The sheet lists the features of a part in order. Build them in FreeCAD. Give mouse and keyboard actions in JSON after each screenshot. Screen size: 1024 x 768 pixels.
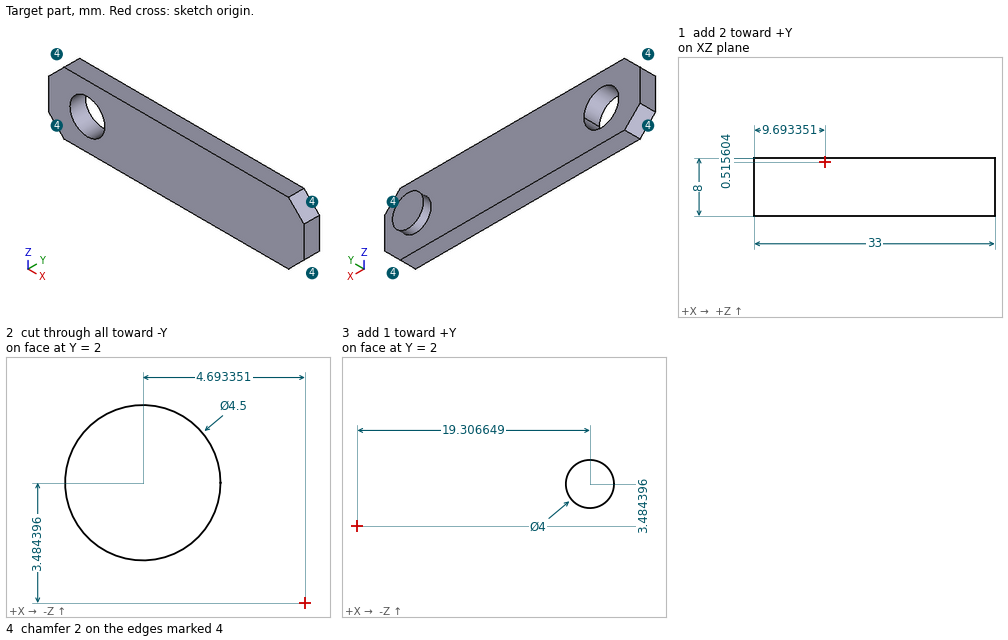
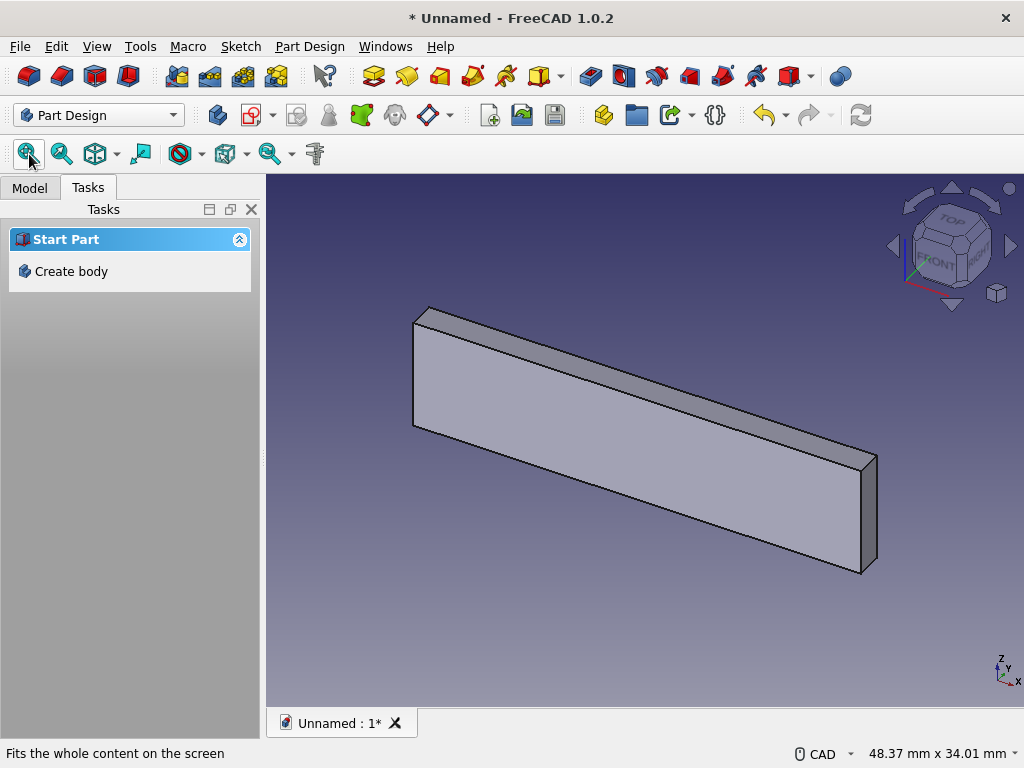
{"action": "key", "text": "4"}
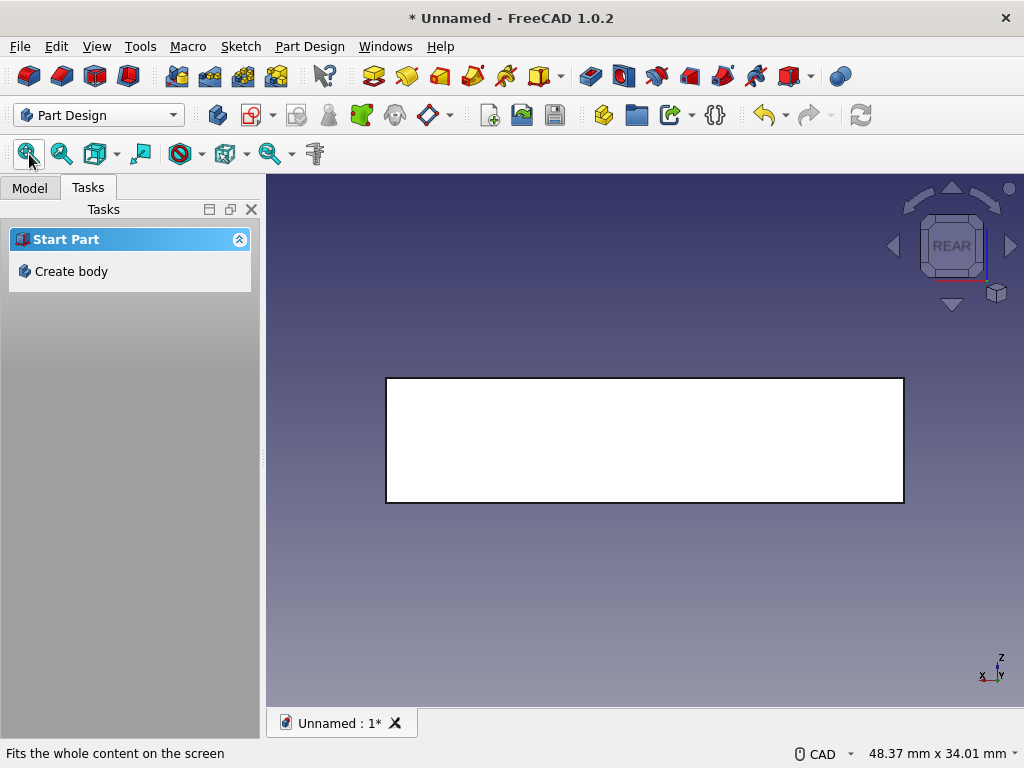
{"action": "left_click", "coordinate": [497, 439]}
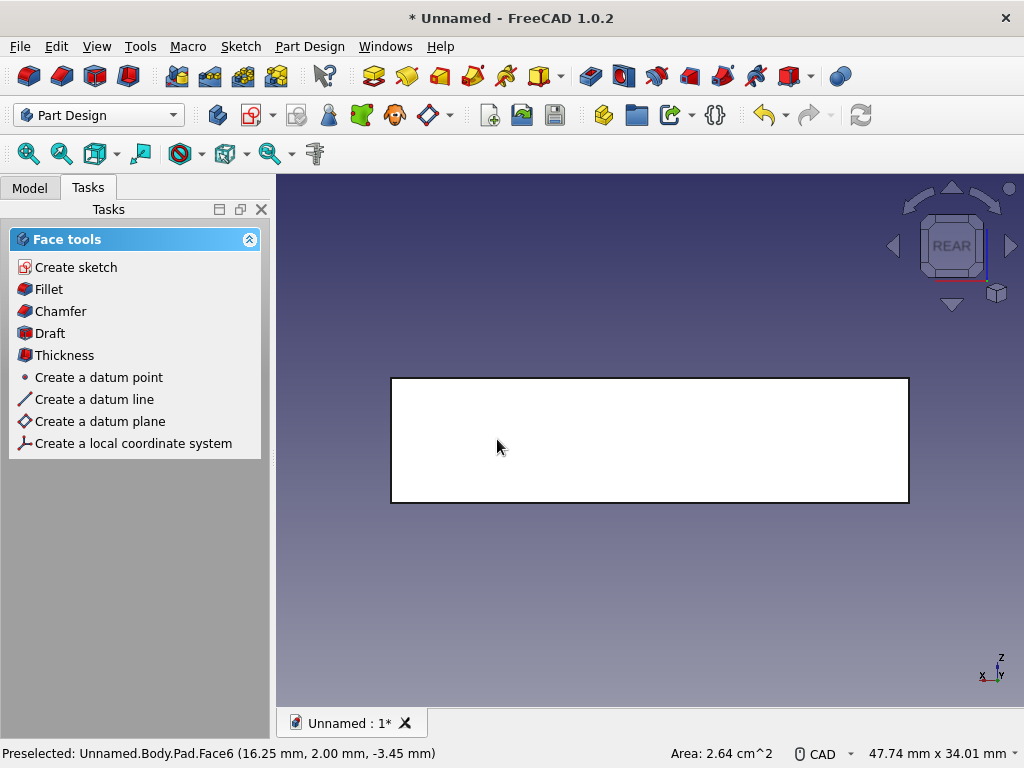
{"action": "left_click", "coordinate": [250, 116]}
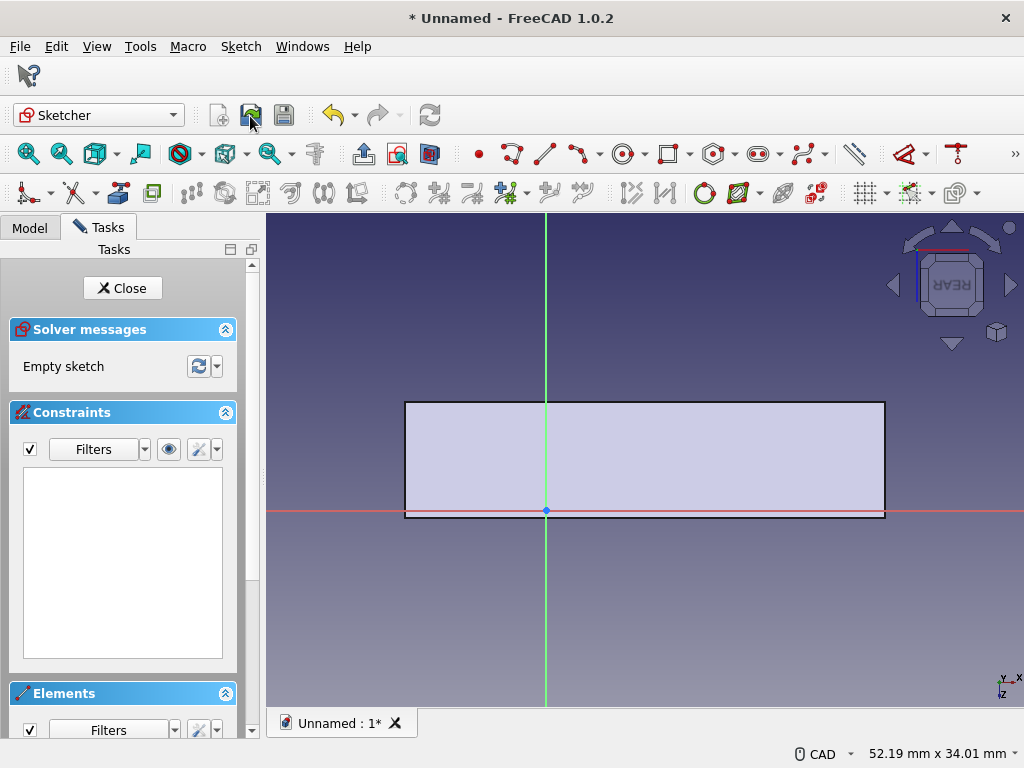
{"action": "scroll", "coordinate": [469, 472], "scroll_direction": "up", "scroll_amount": 7}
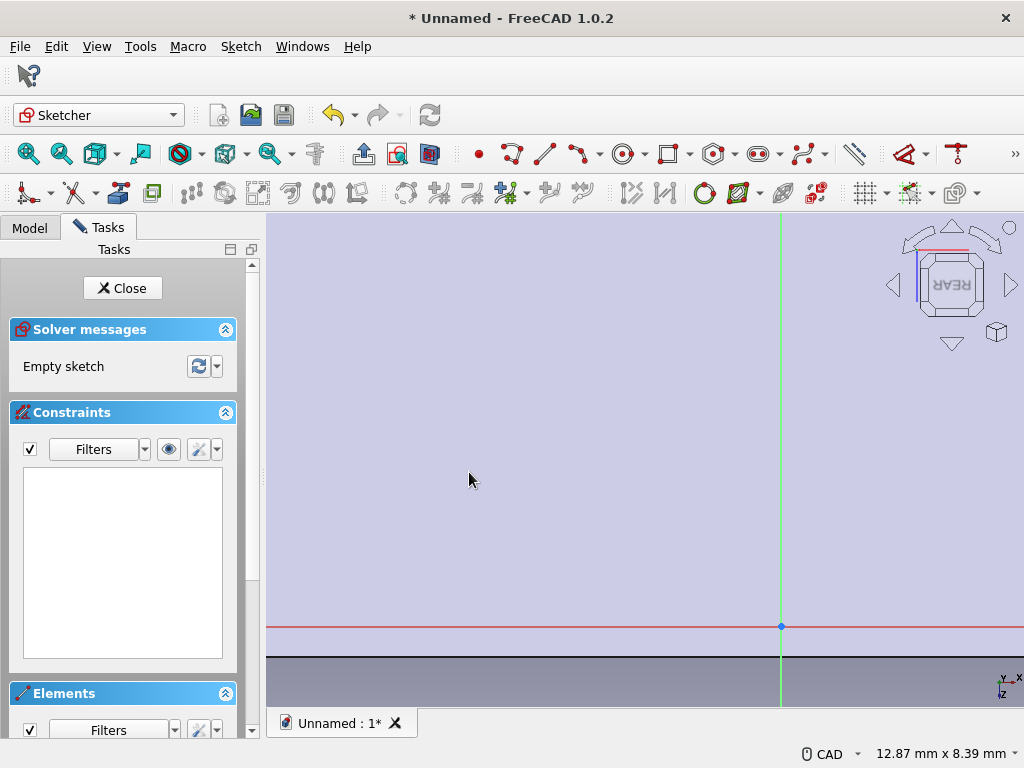
{"action": "left_click", "coordinate": [622, 154]}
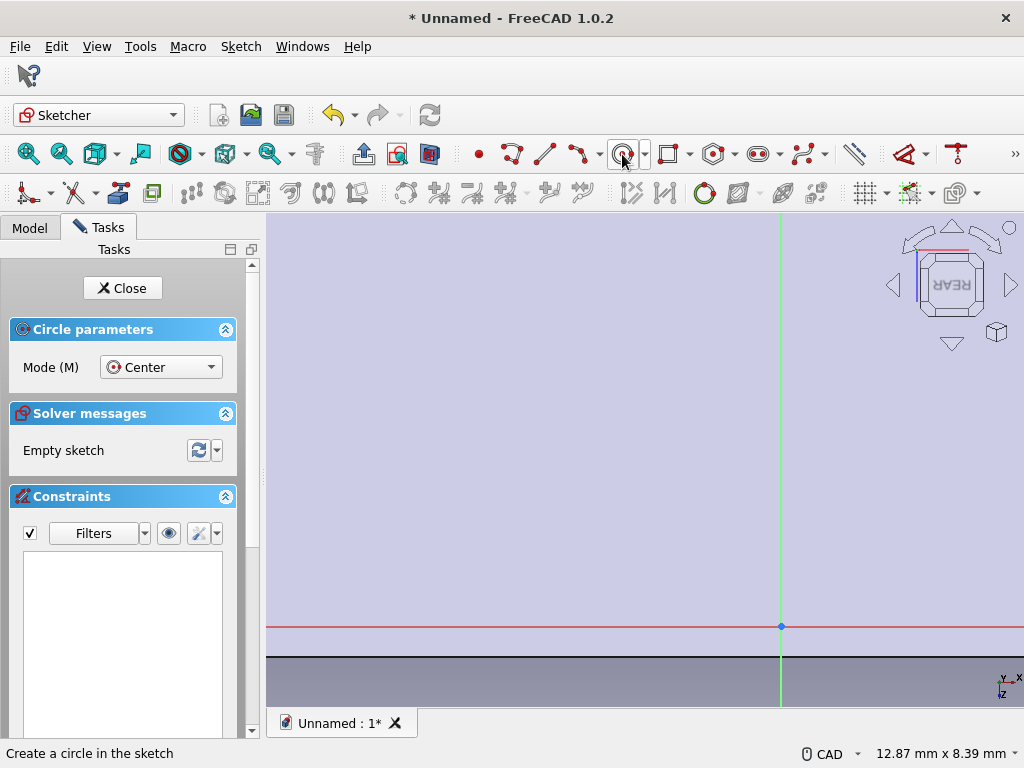
{"action": "left_click", "coordinate": [505, 422]}
{"action": "left_click", "coordinate": [598, 328]}
{"action": "key", "text": "Escape"}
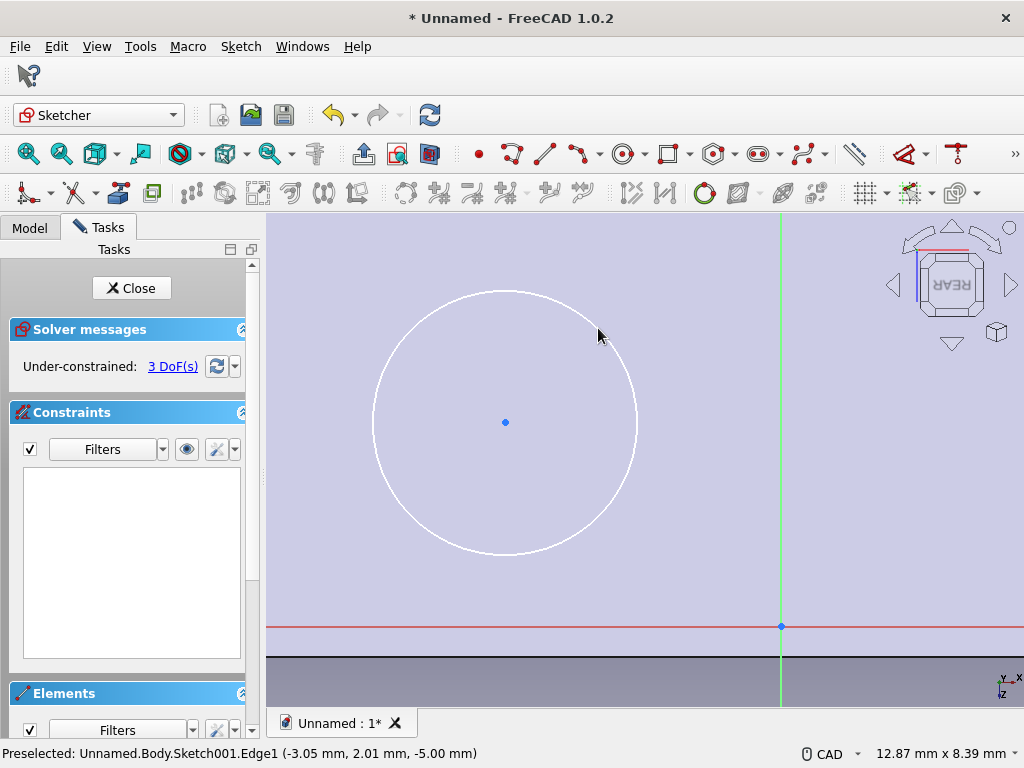
{"action": "left_click", "coordinate": [904, 154]}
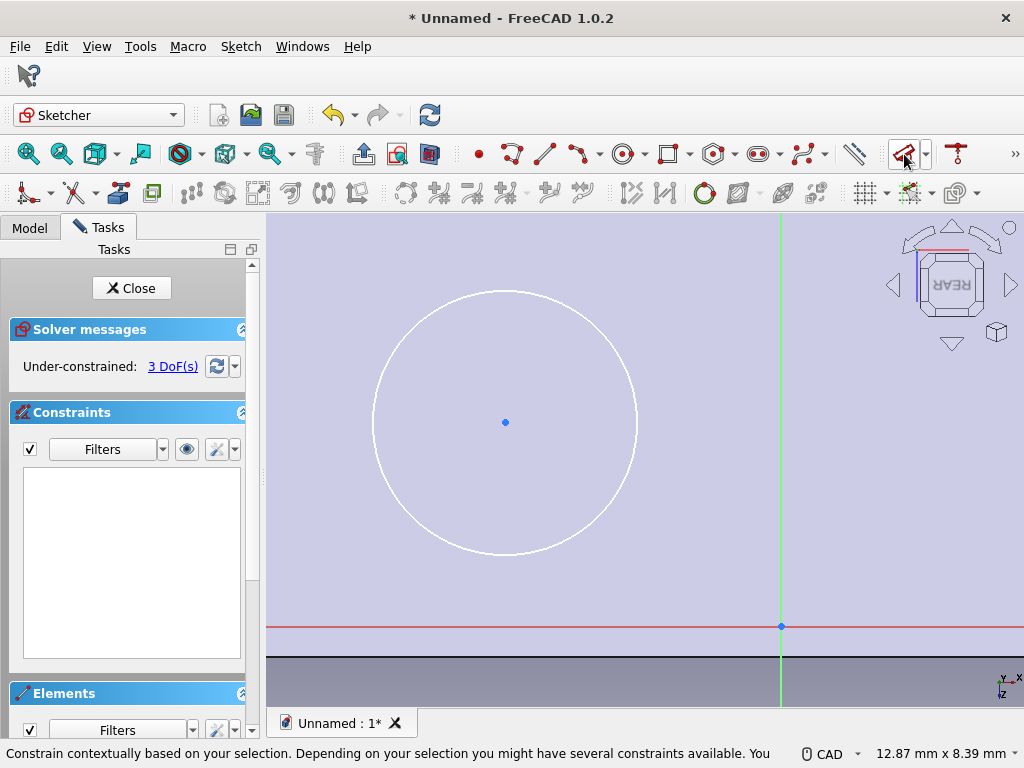
{"action": "left_click", "coordinate": [598, 329]}
{"action": "left_click", "coordinate": [621, 306]}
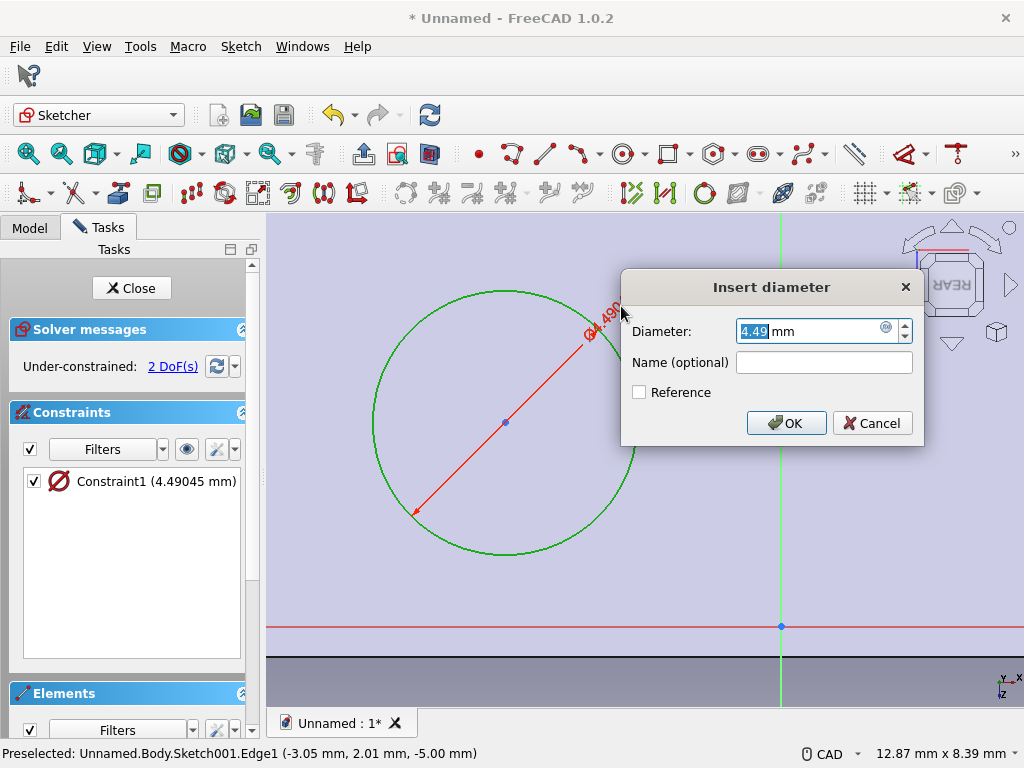
{"action": "type", "text": "4.5"}
{"action": "key", "text": "Return"}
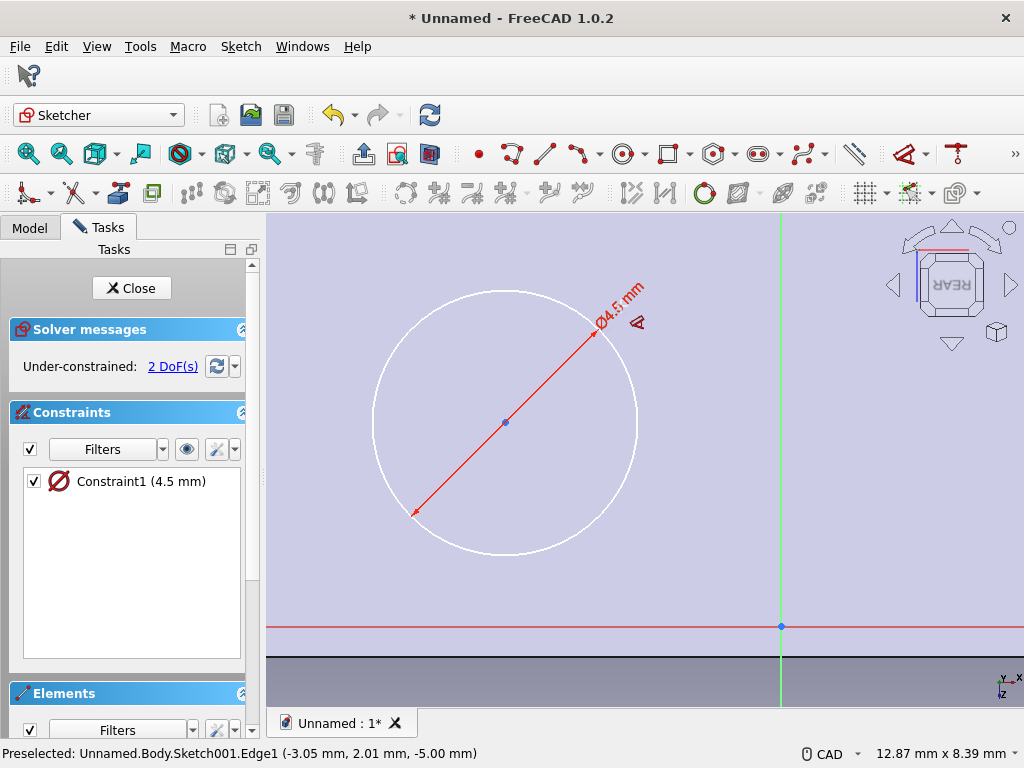
{"action": "left_click", "coordinate": [505, 423]}
{"action": "left_click", "coordinate": [643, 661]}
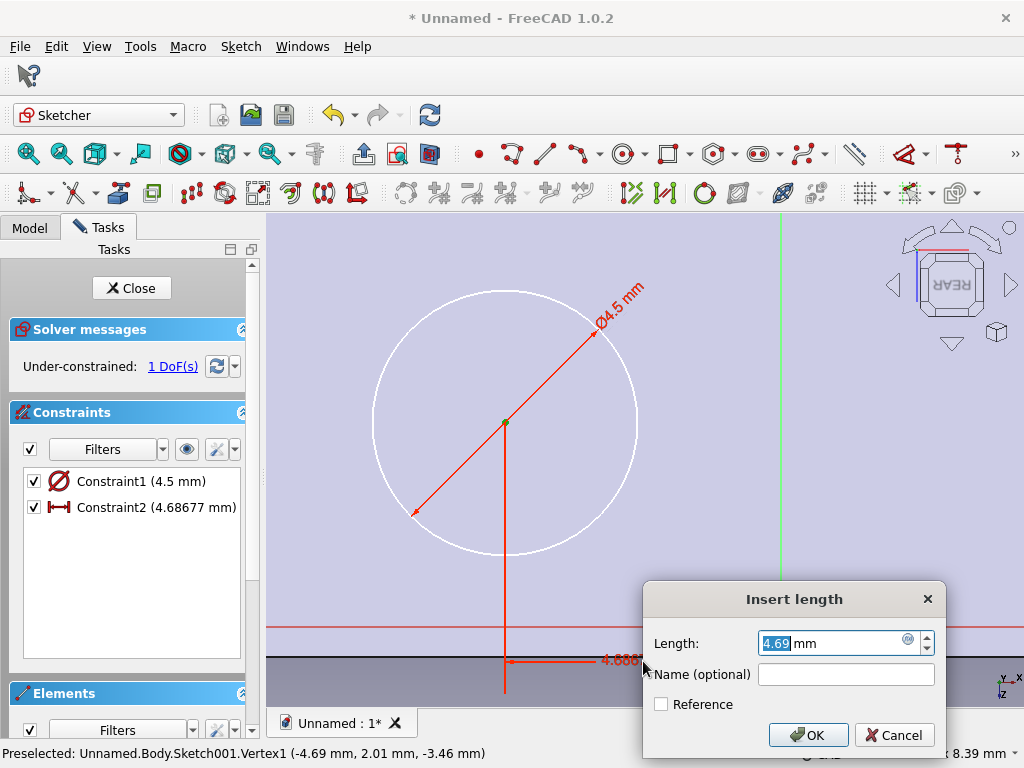
{"action": "type", "text": "4.693351"}
{"action": "key", "text": "Return"}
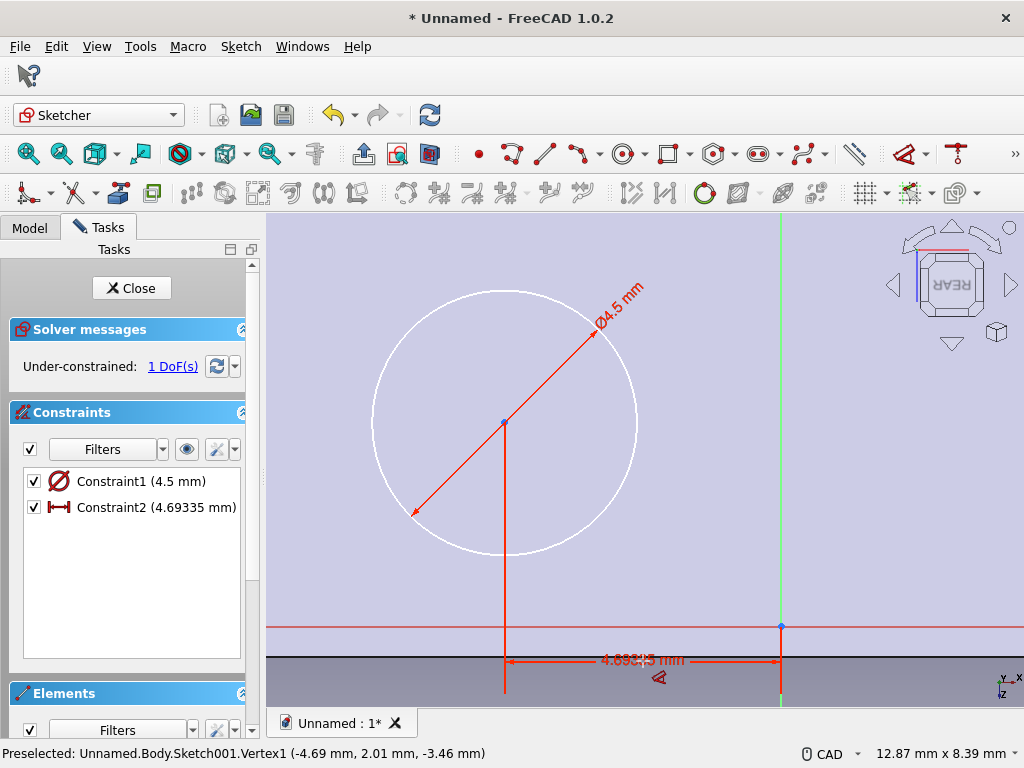
{"action": "left_click", "coordinate": [505, 423]}
{"action": "left_click", "coordinate": [815, 525]}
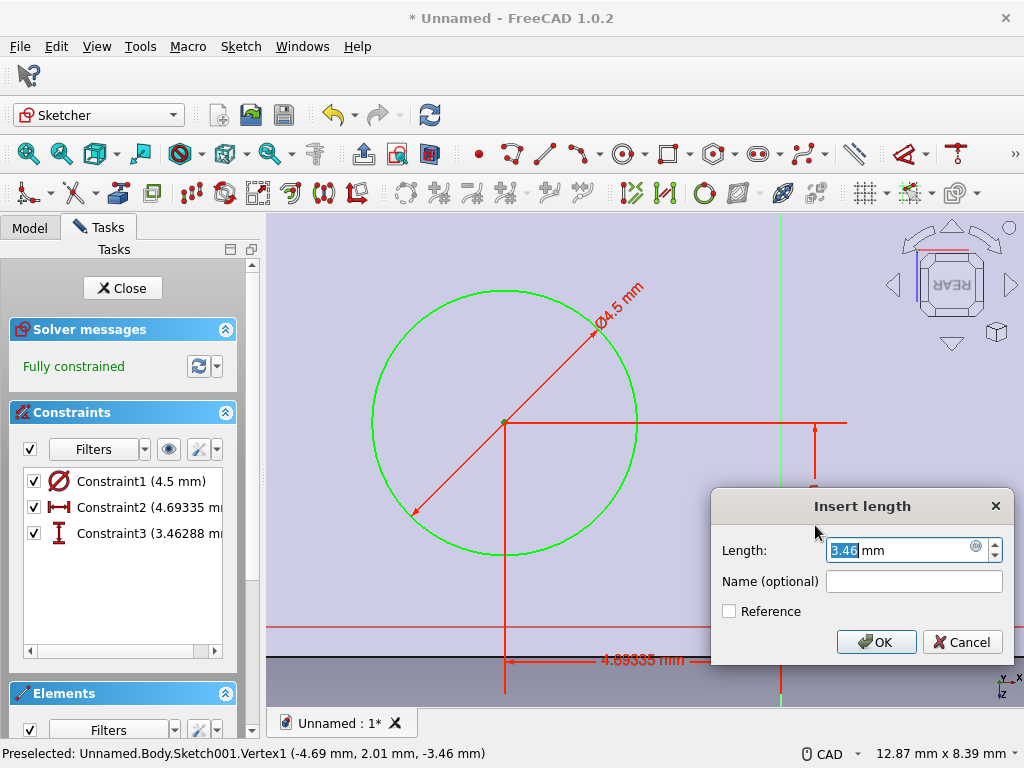
{"action": "type", "text": "3.484396"}
{"action": "key", "text": "Return"}
{"action": "key", "text": "Escape"}